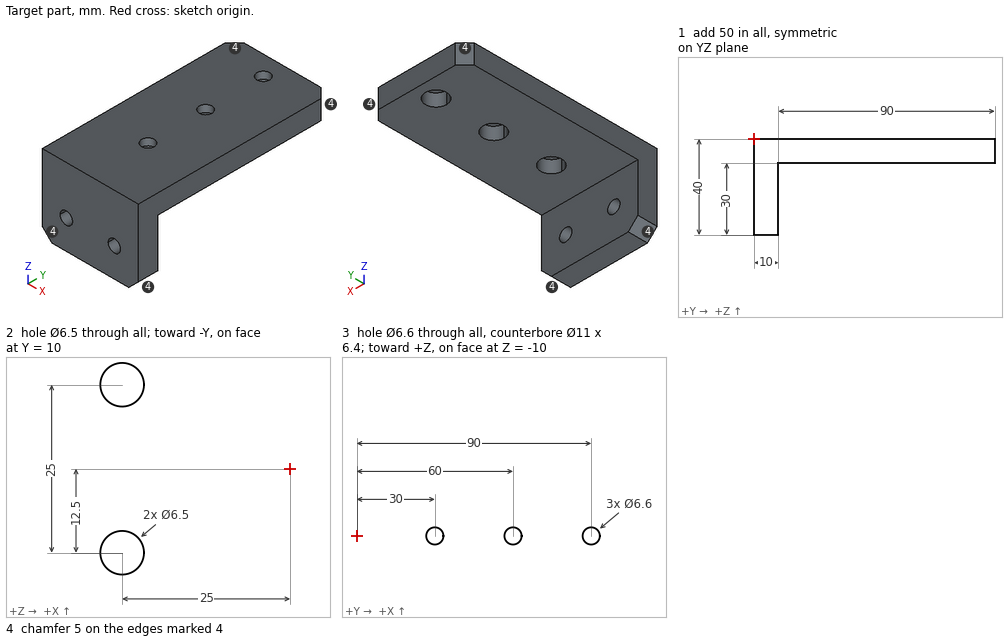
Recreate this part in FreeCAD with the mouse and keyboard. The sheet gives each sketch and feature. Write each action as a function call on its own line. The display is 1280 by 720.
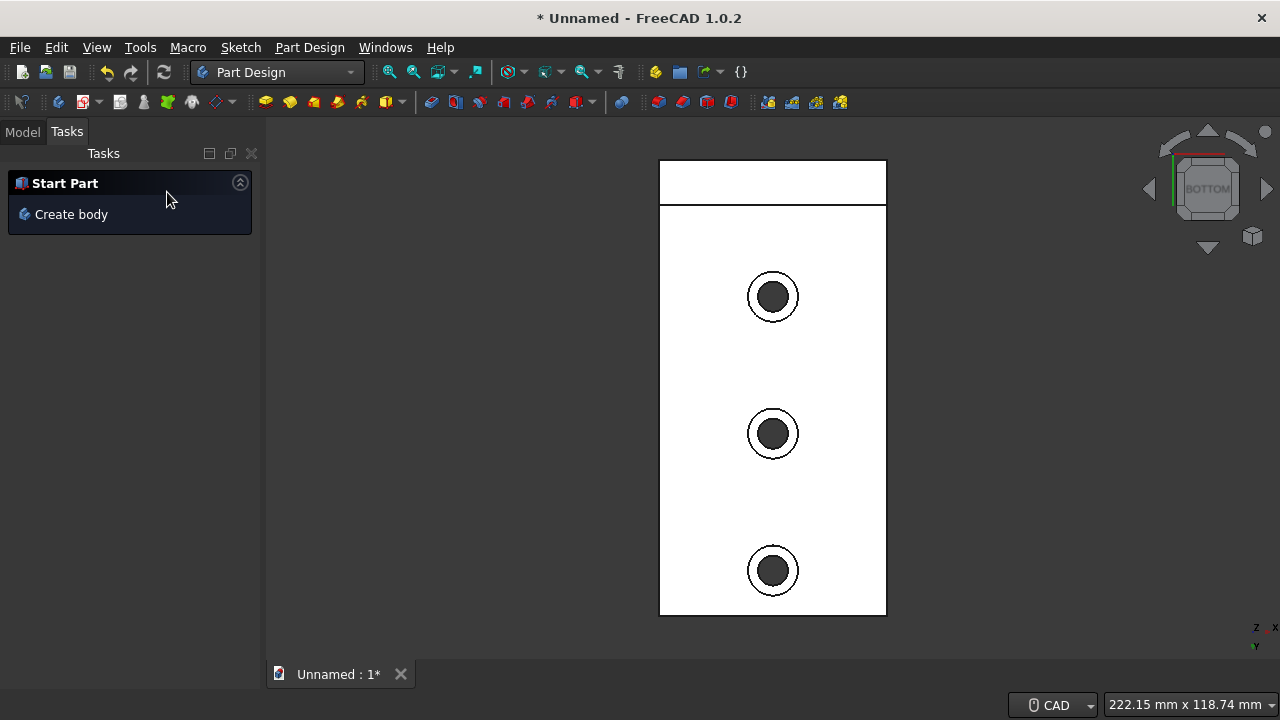
click(659, 182)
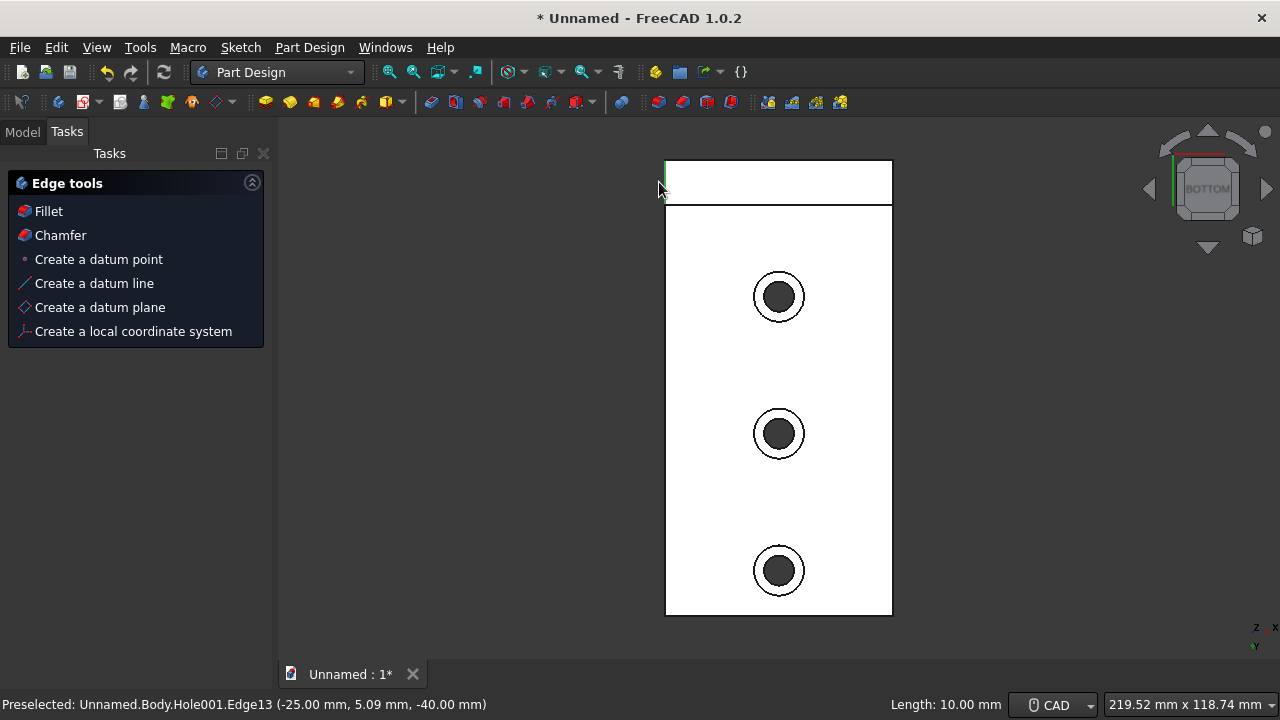
click(893, 182, ctrl)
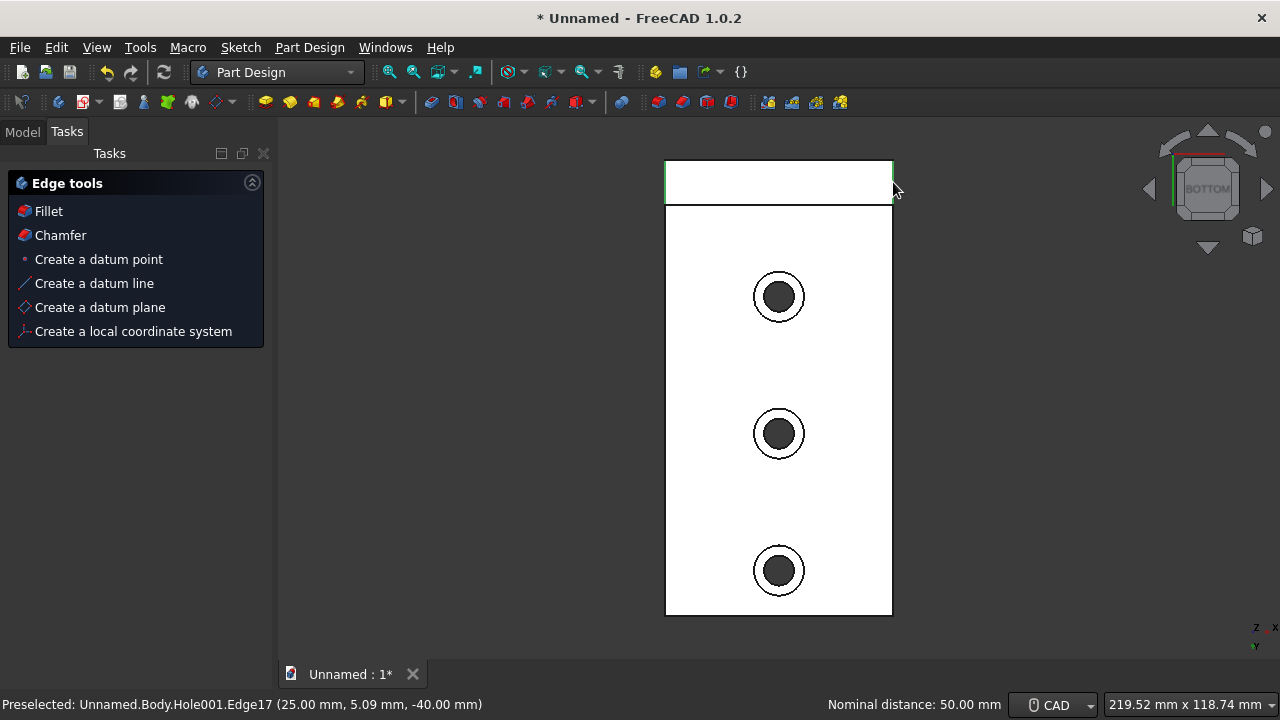
key(0)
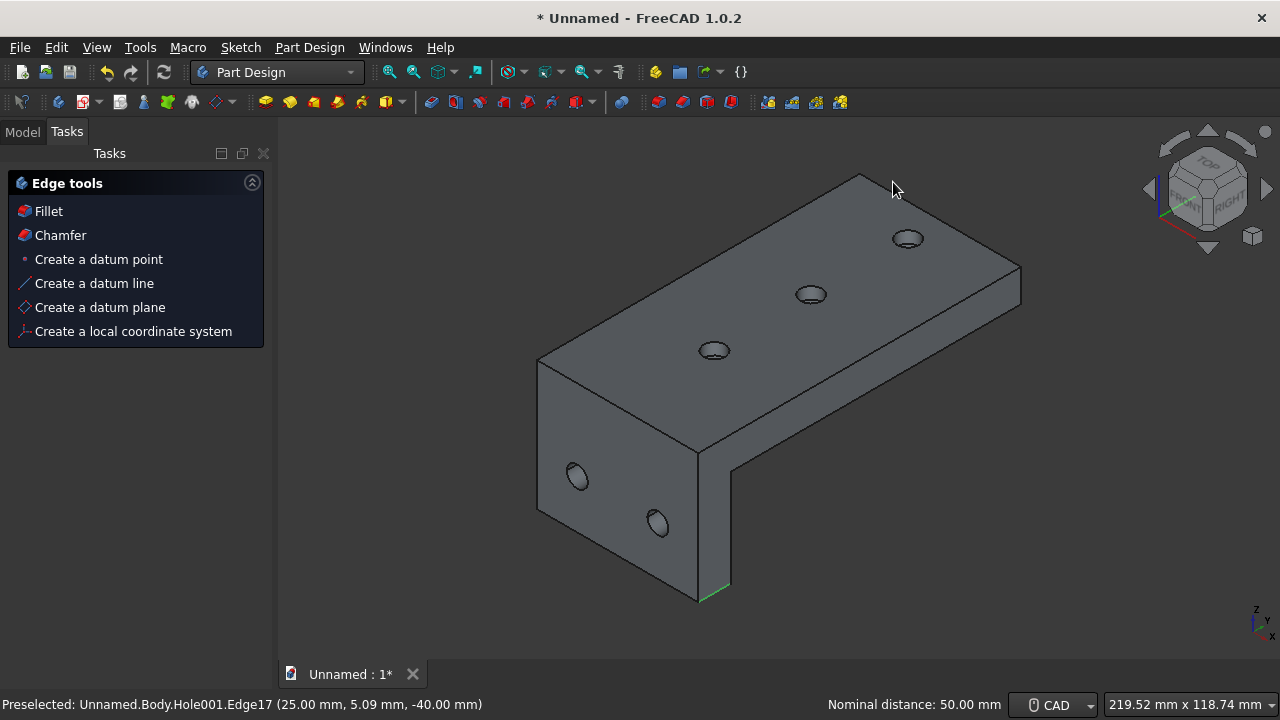
key(2)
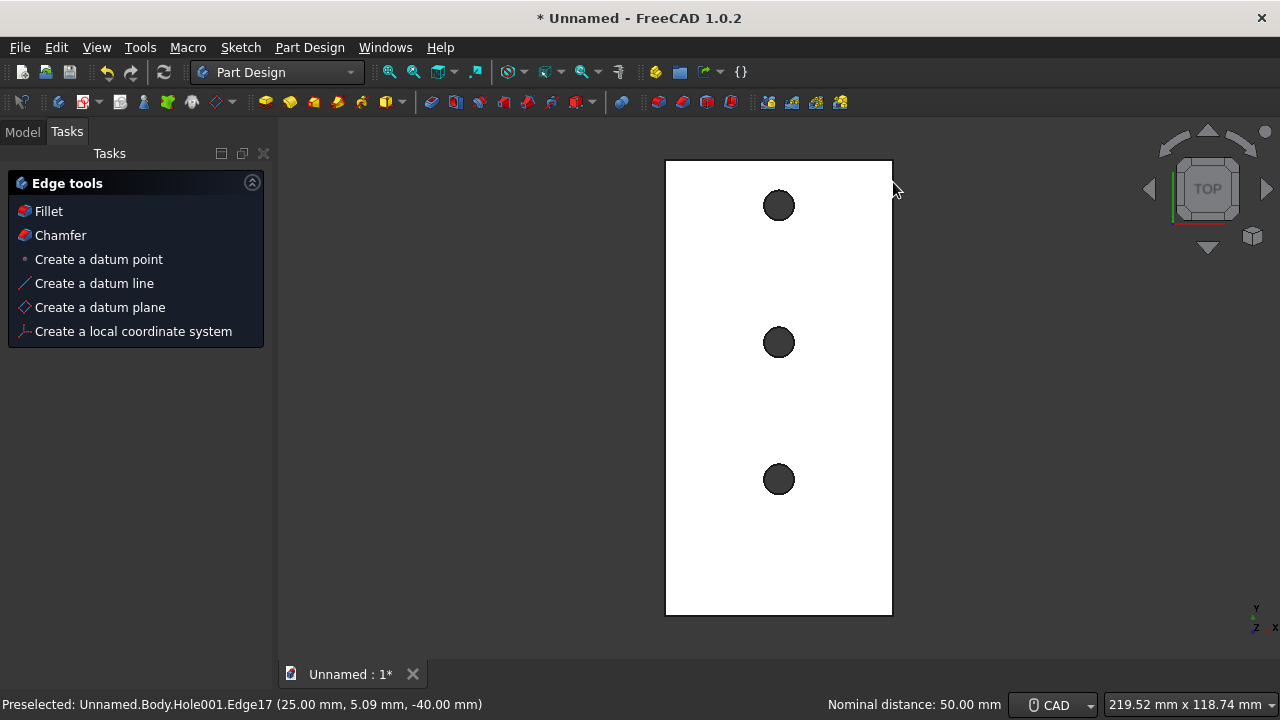
key(1)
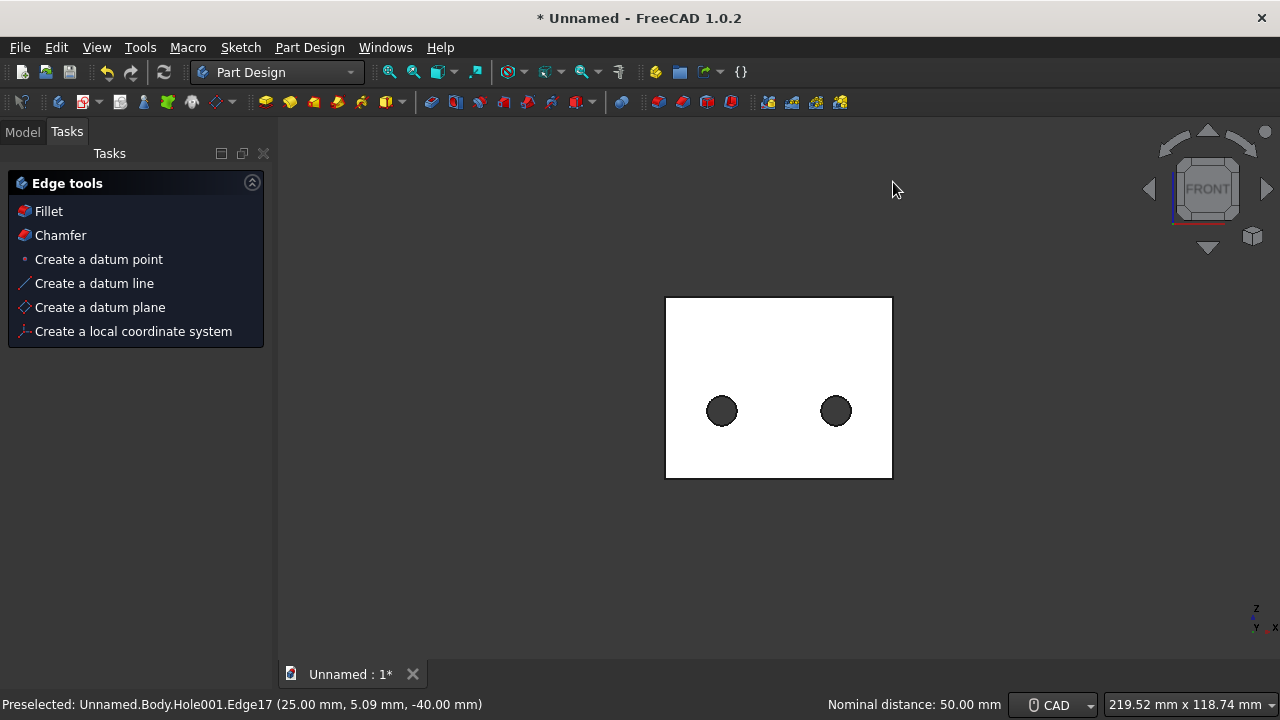
click(390, 72)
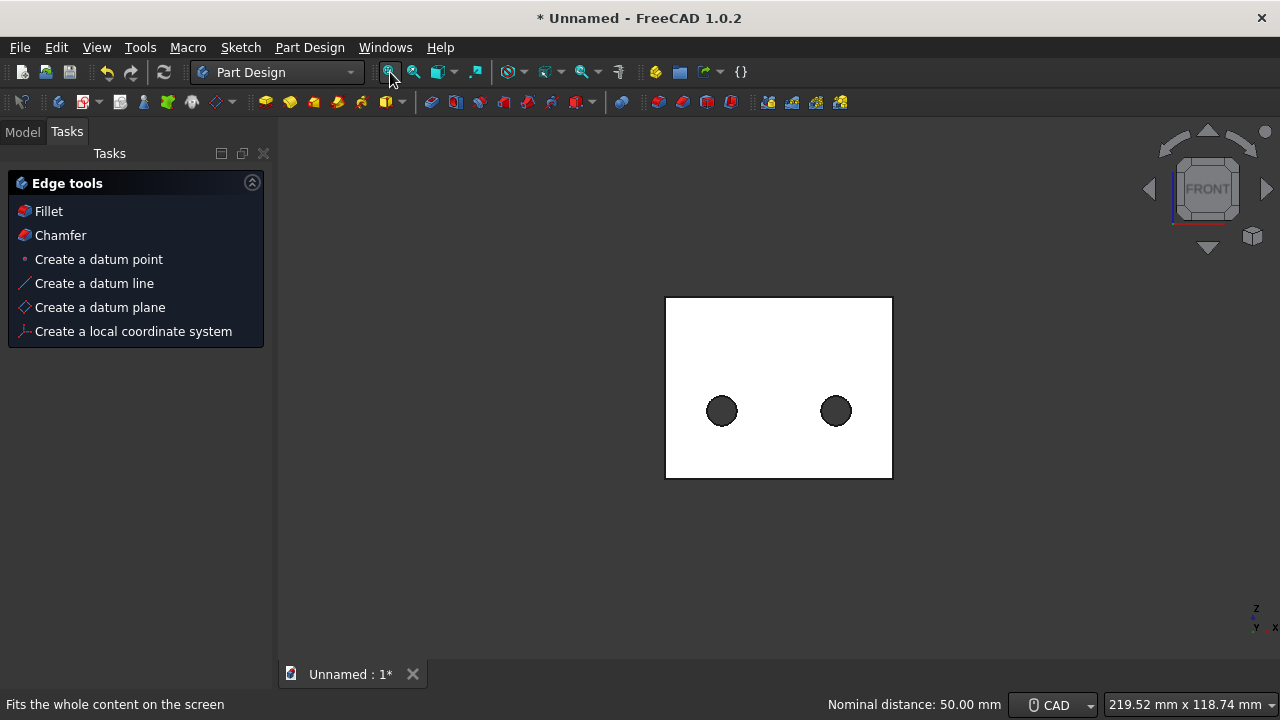
key(3)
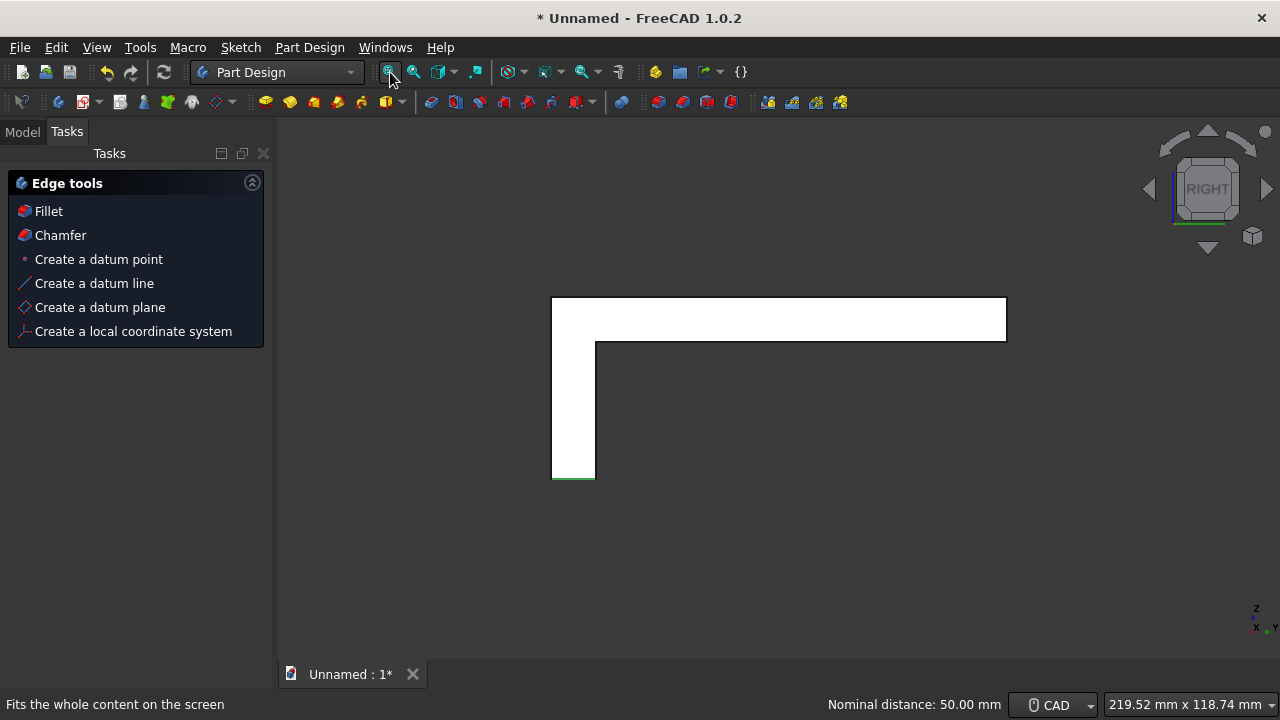
click(1007, 319, ctrl)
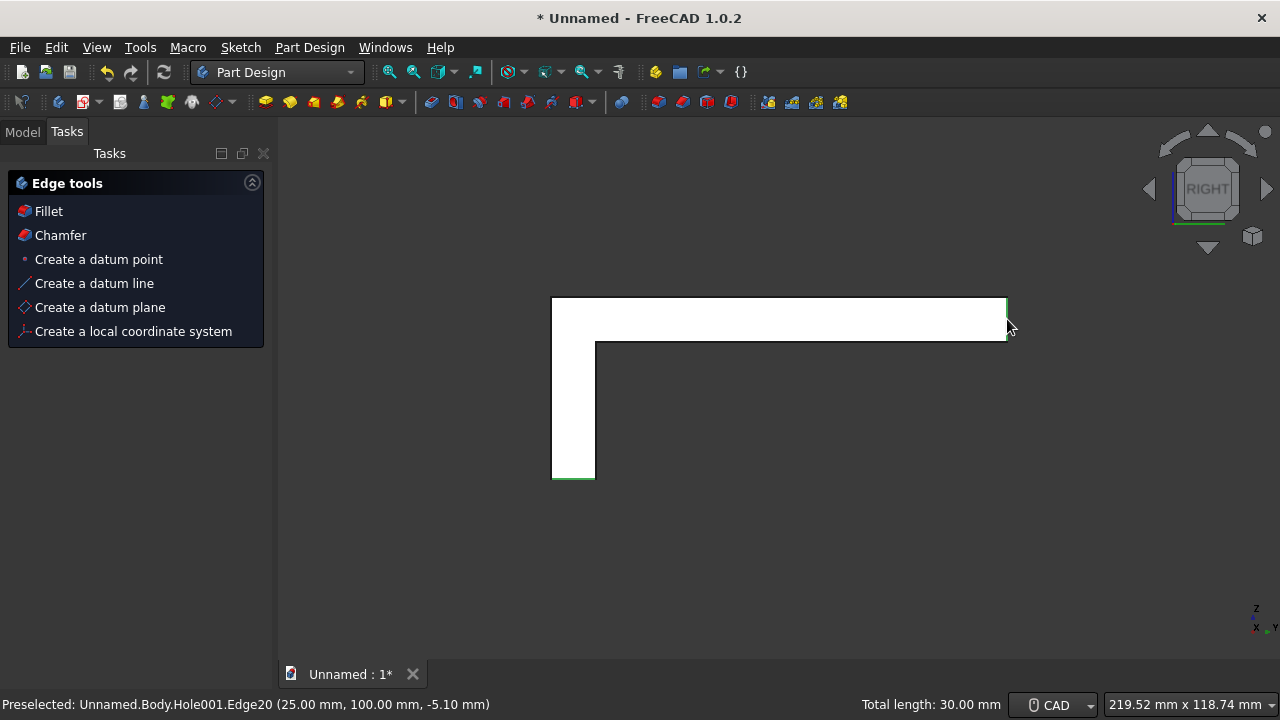
key(5)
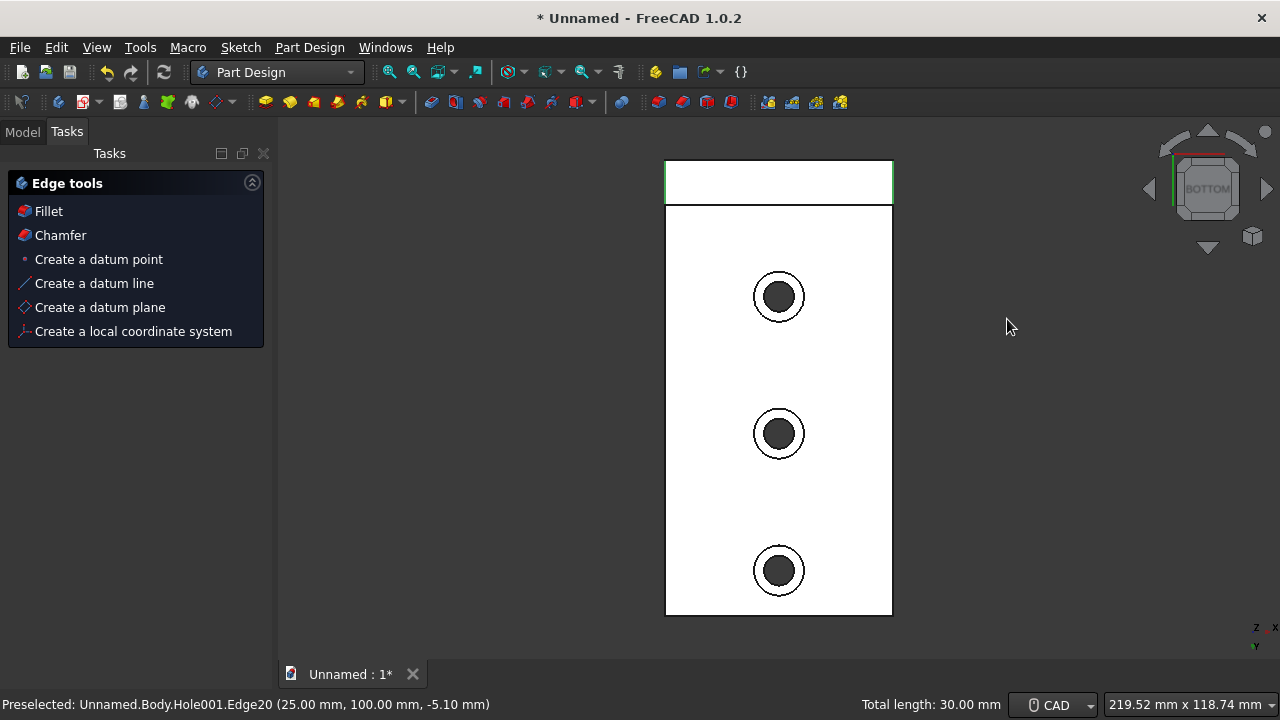
key(4)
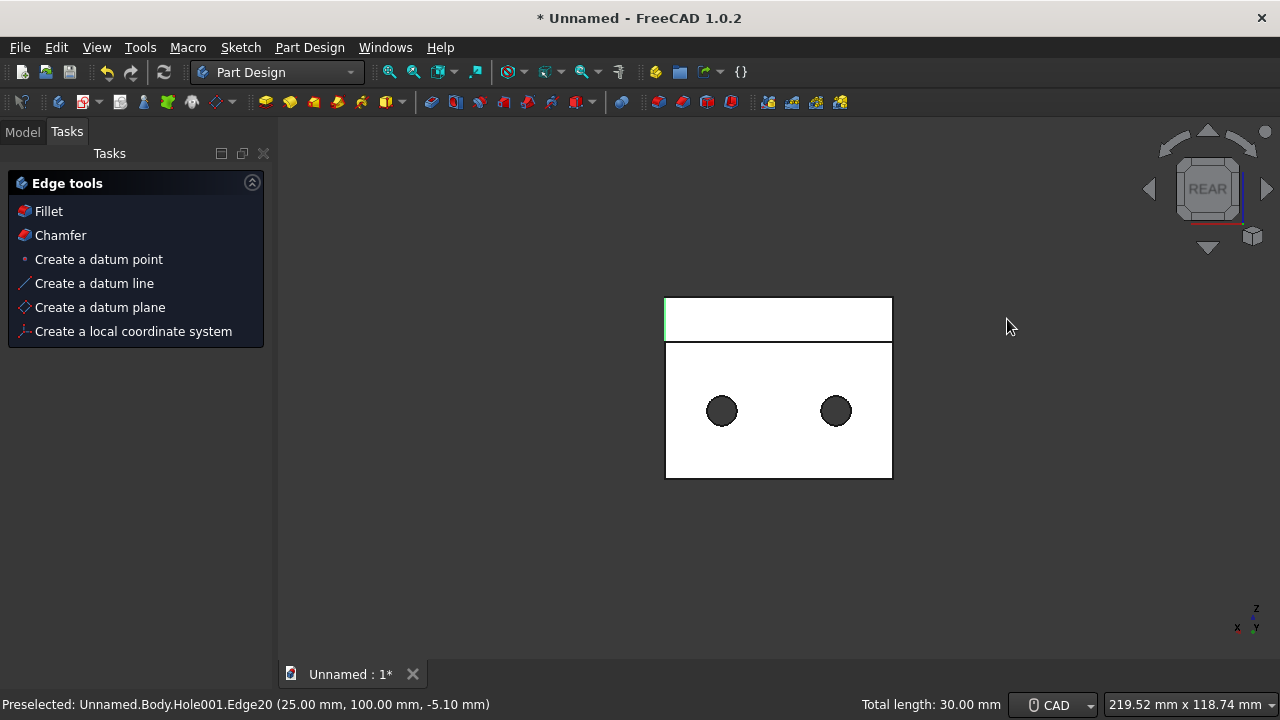
click(390, 72)